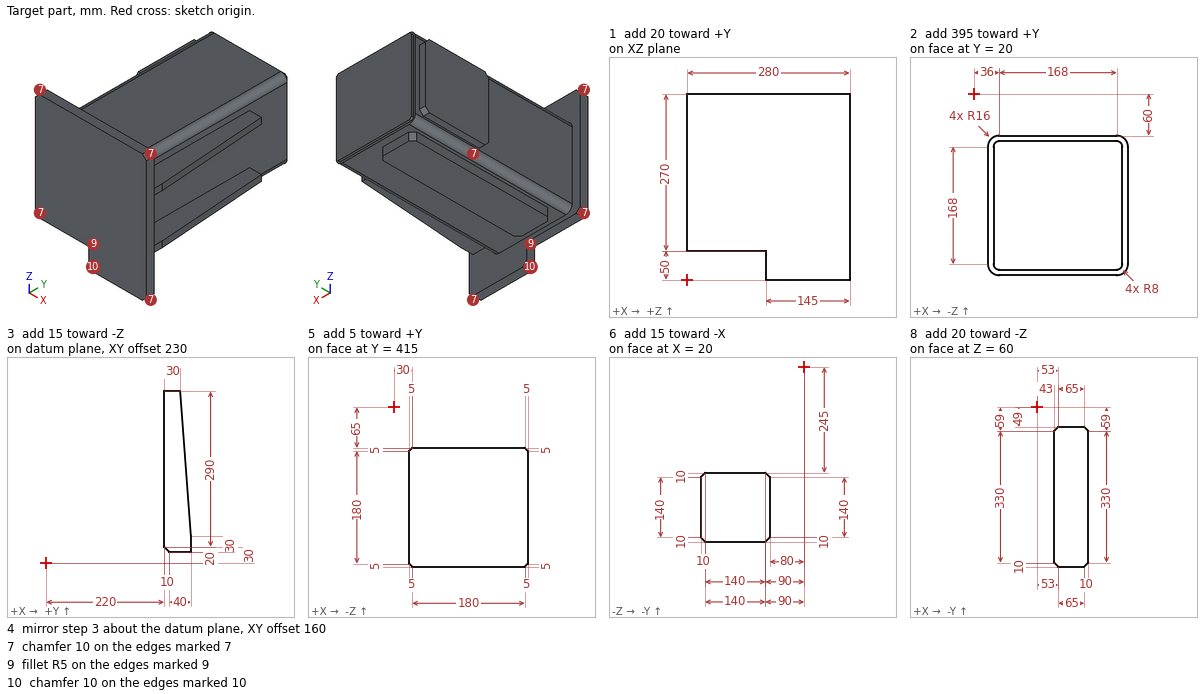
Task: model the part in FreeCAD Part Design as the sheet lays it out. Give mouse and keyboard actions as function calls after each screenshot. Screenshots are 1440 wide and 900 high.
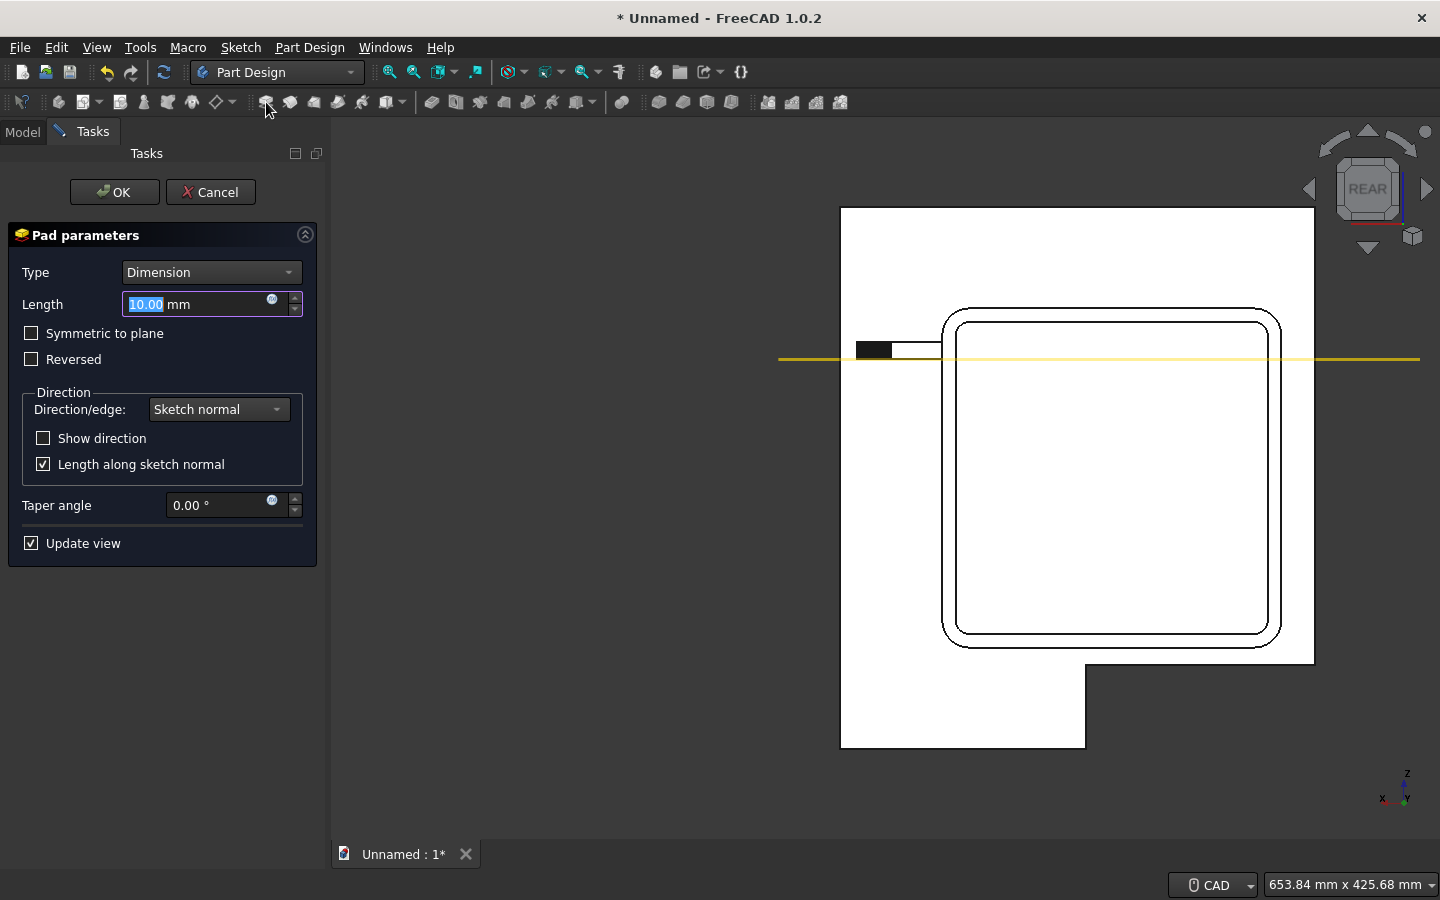
text(15)
key(Tab)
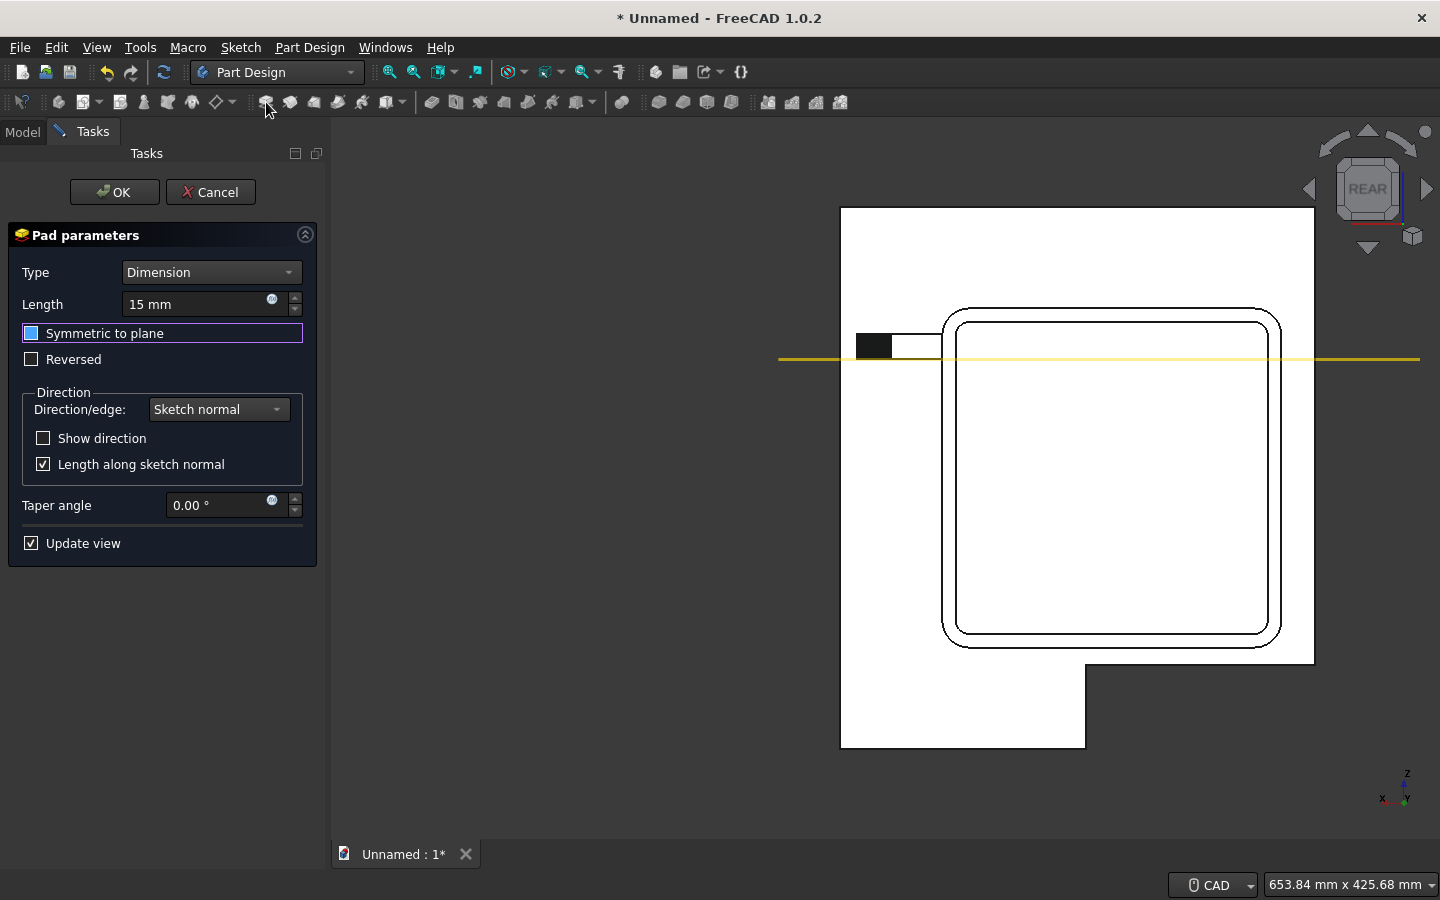
click(30, 359)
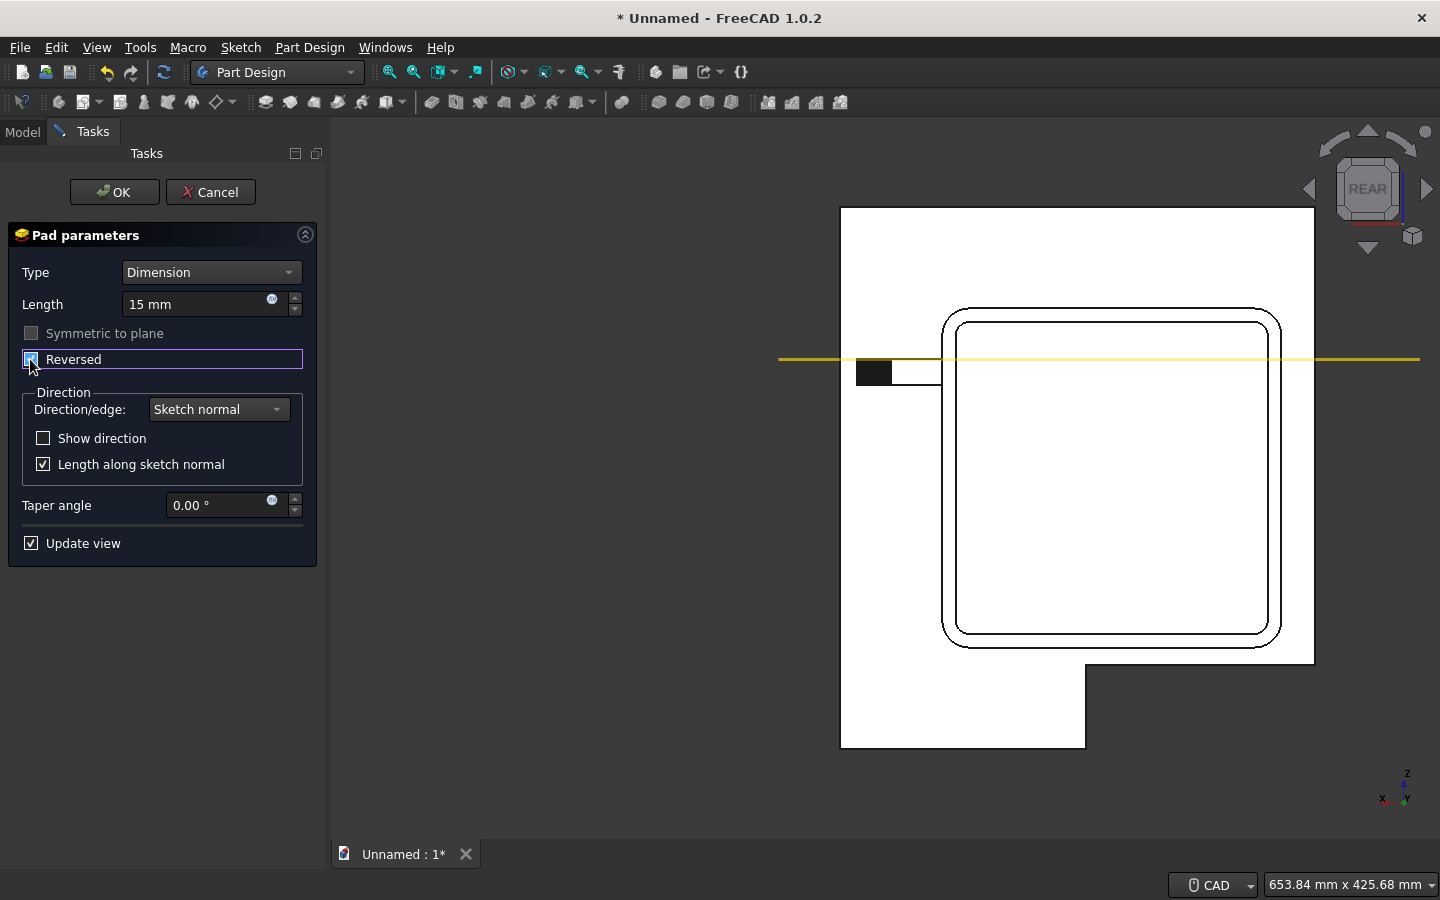
click(115, 192)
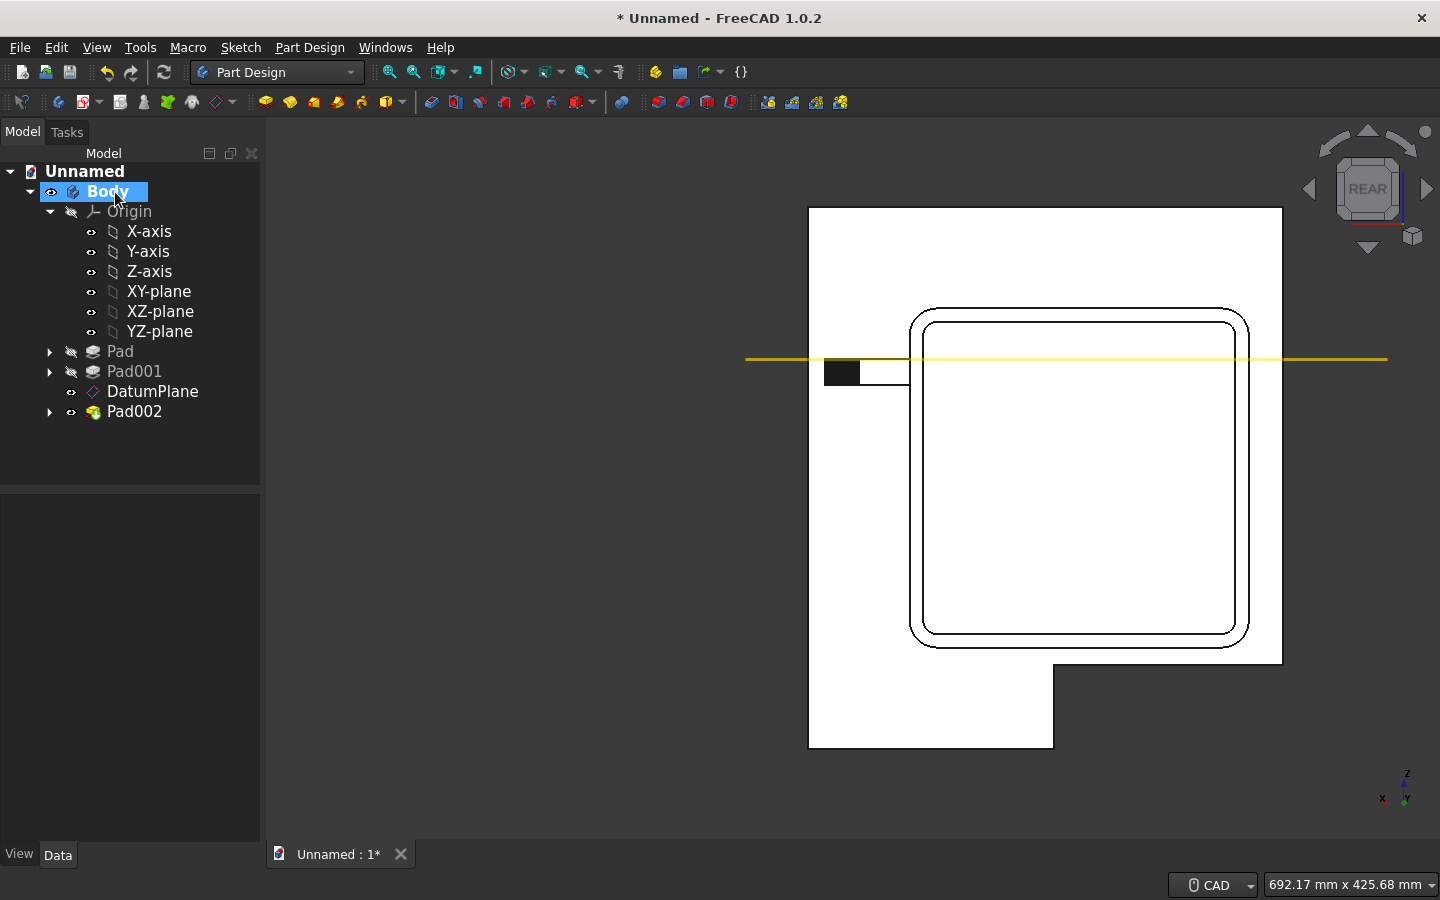
click(116, 392)
key(space)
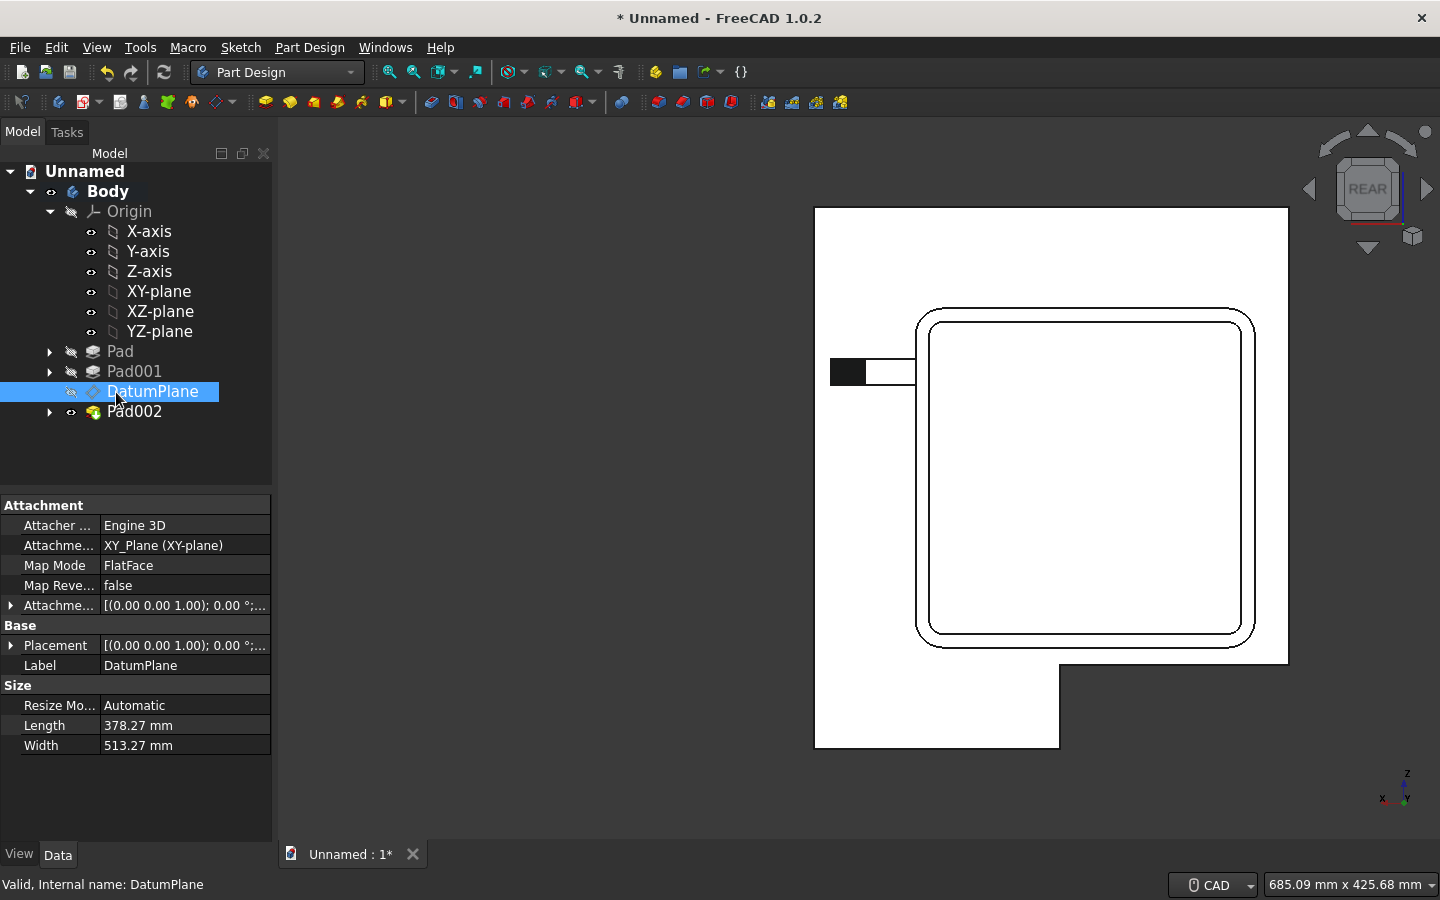
click(136, 292)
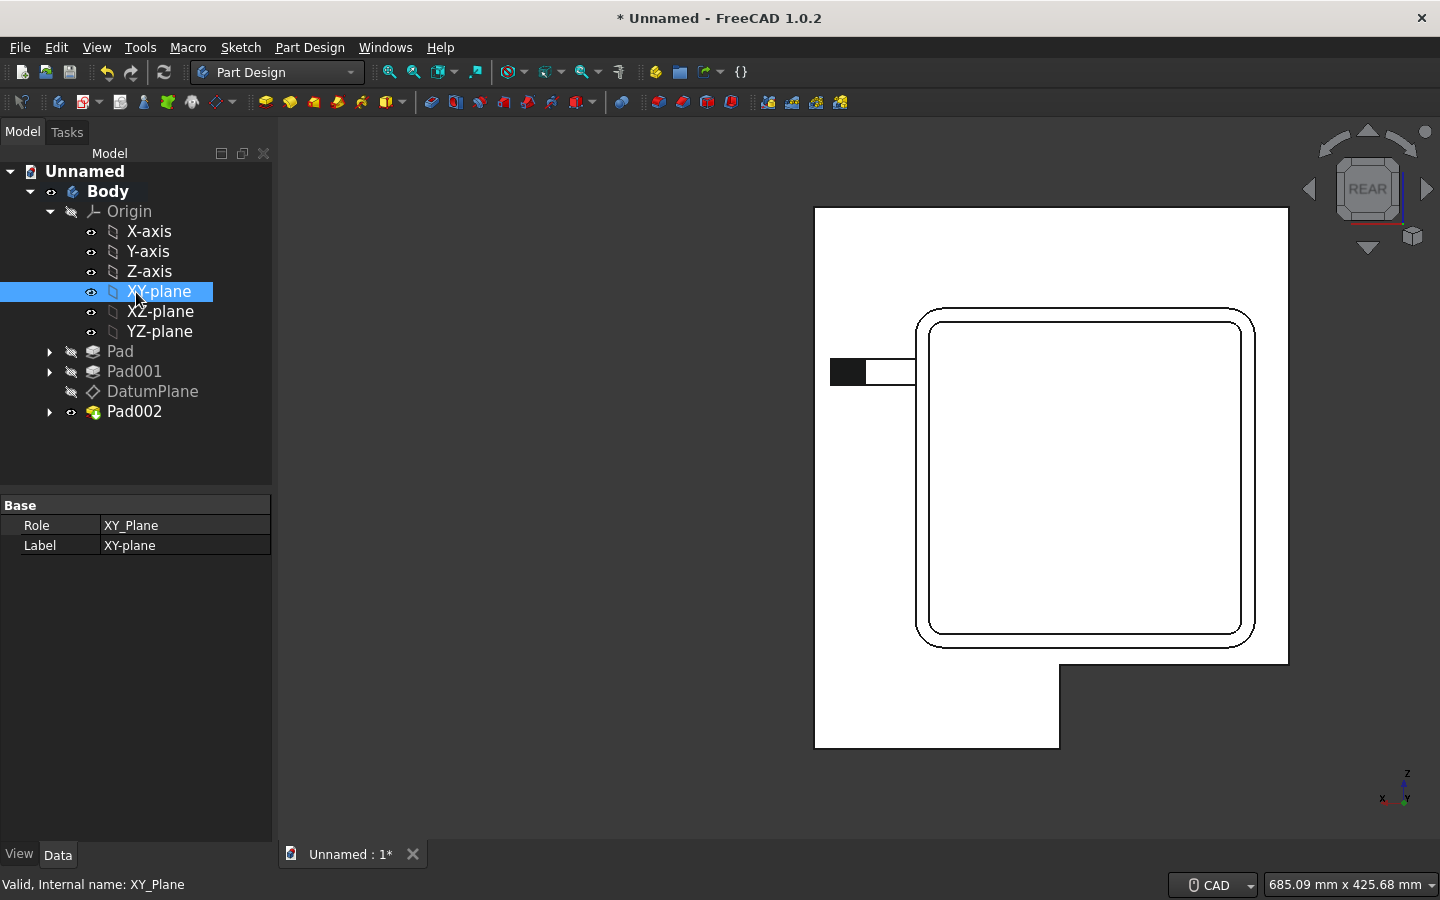
click(216, 102)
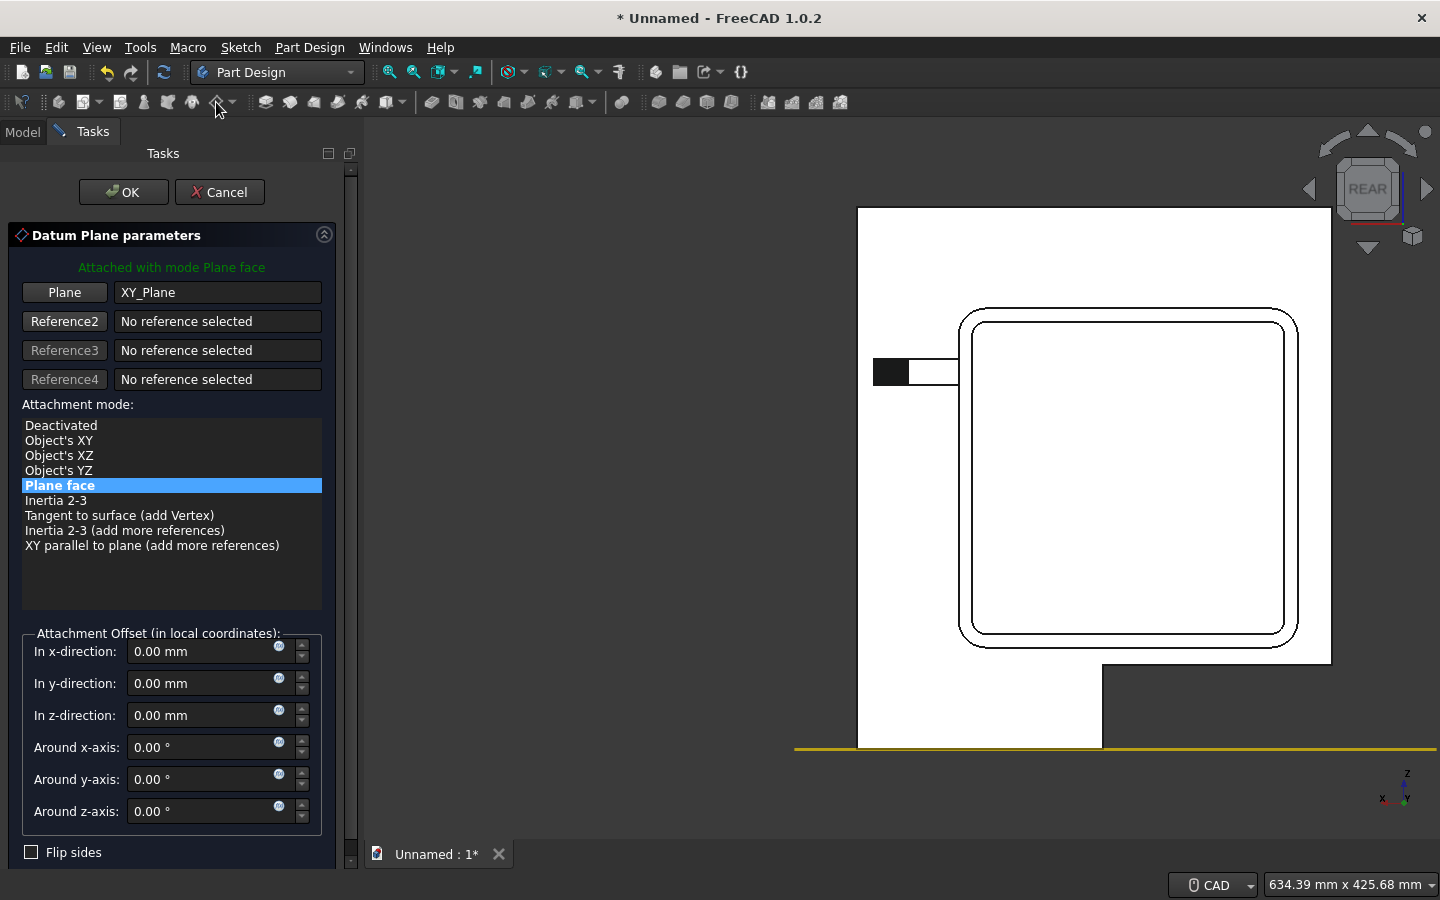
triple_click(210, 715)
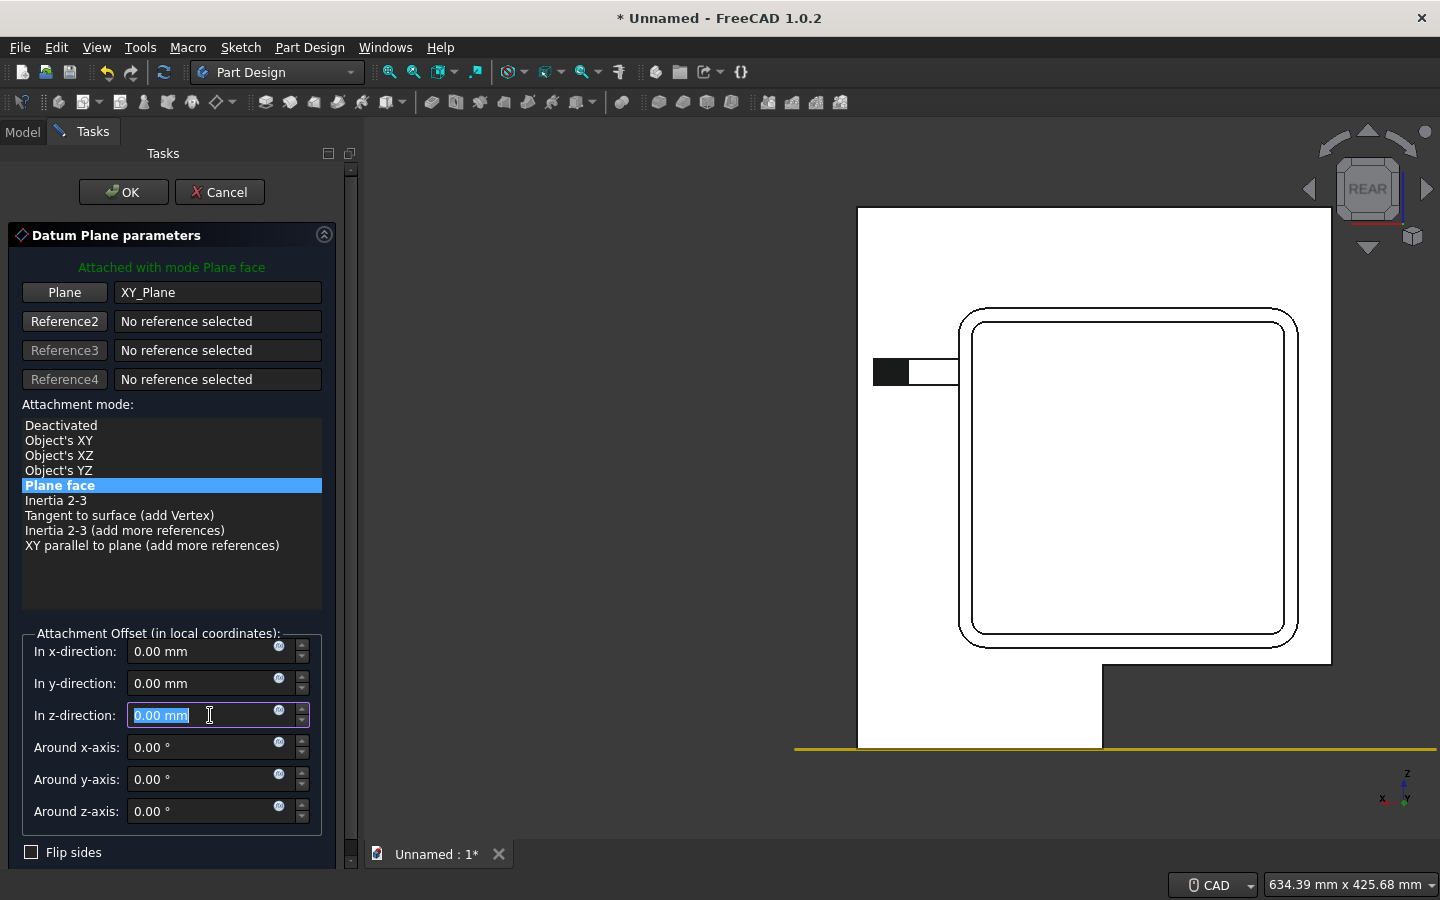
text(160)
key(Tab)